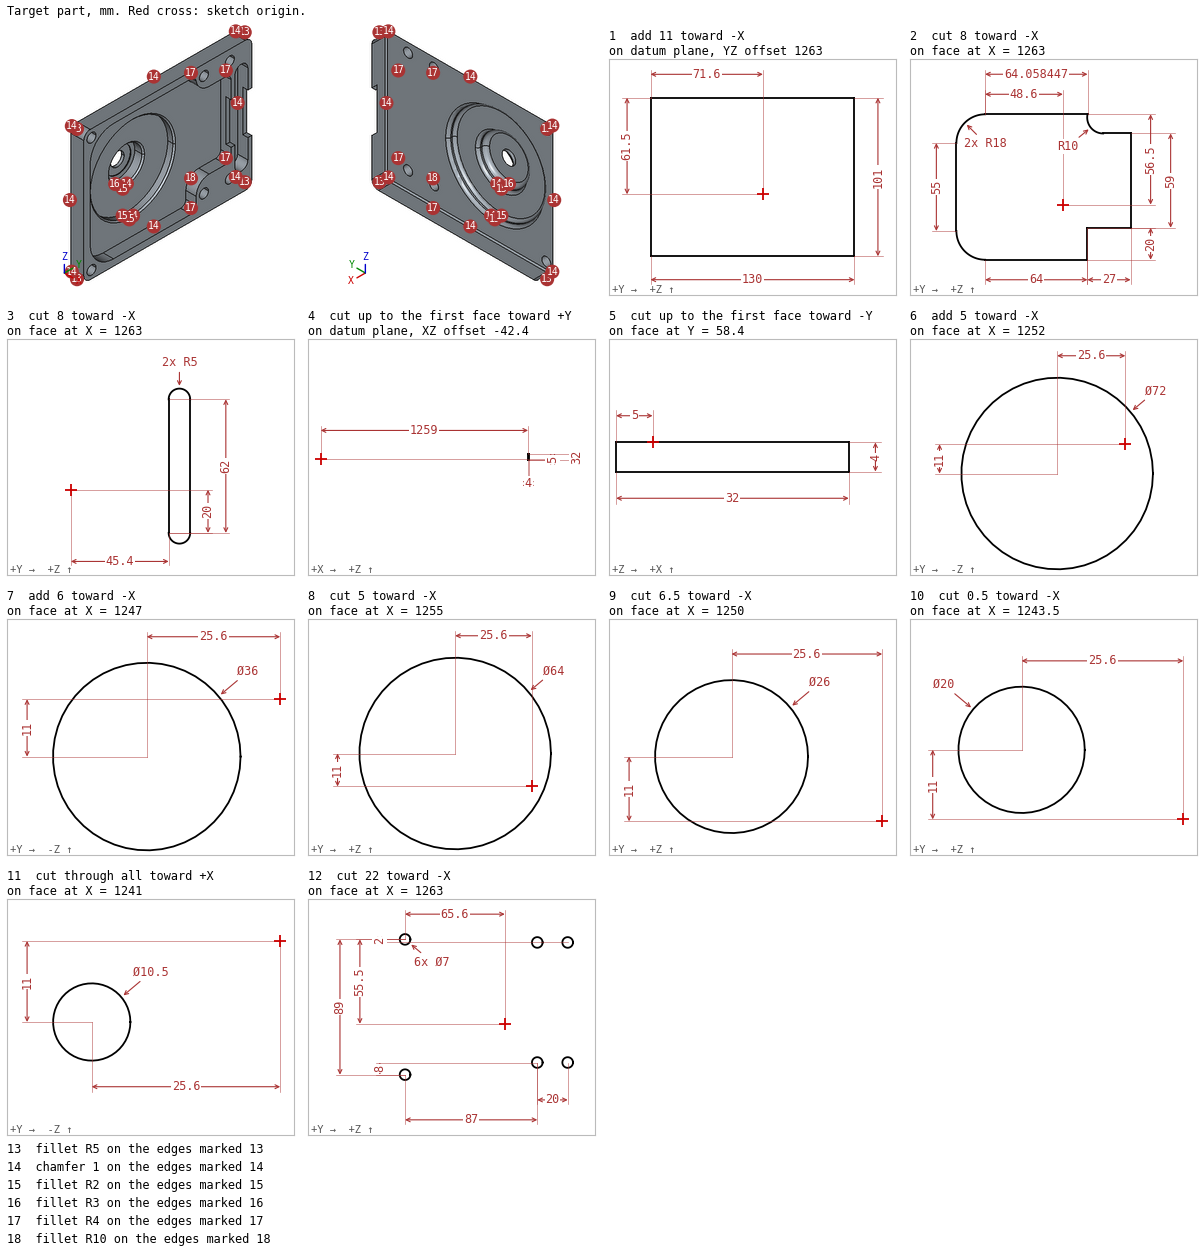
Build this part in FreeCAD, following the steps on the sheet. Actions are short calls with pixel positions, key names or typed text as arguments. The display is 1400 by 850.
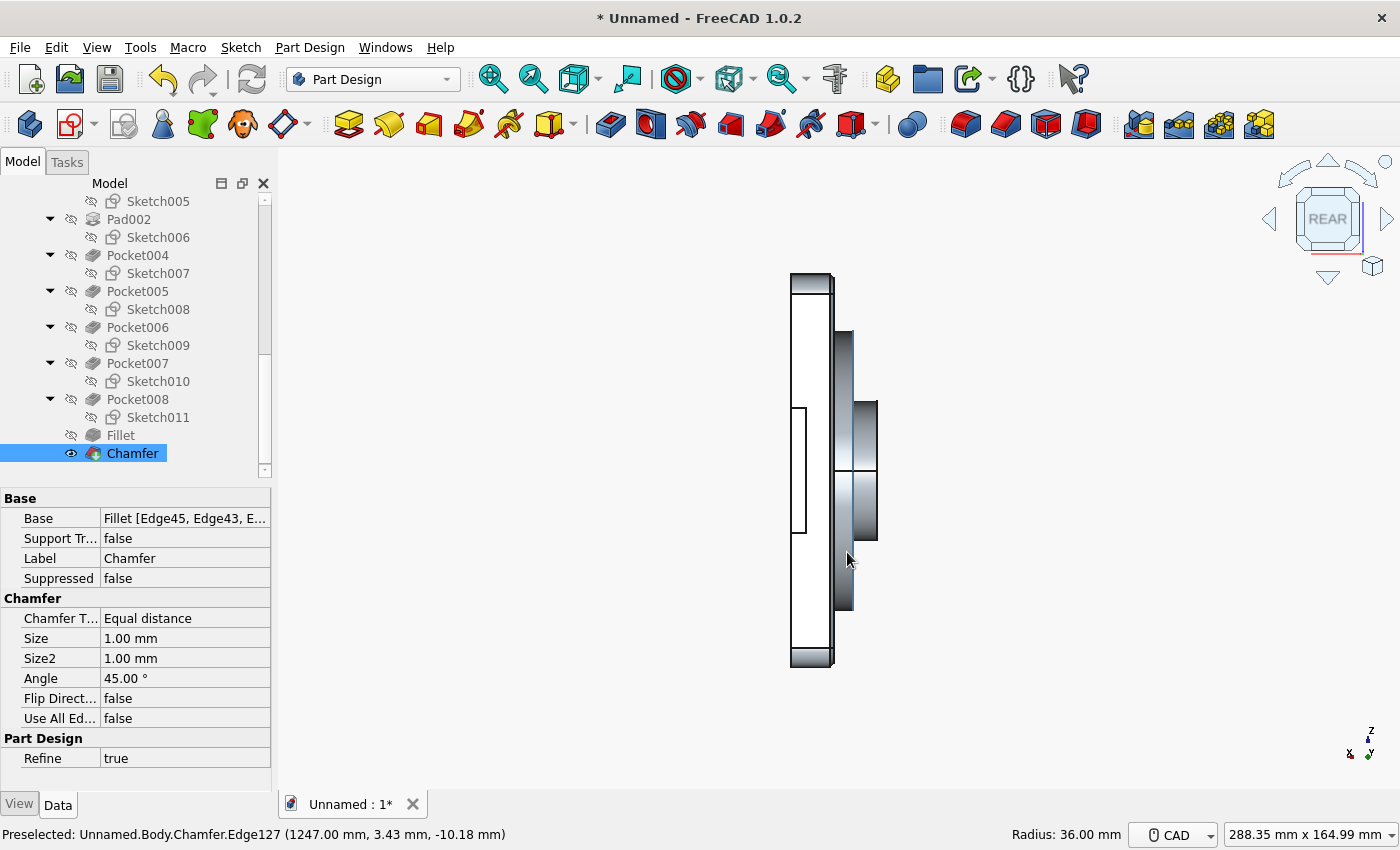
key(6)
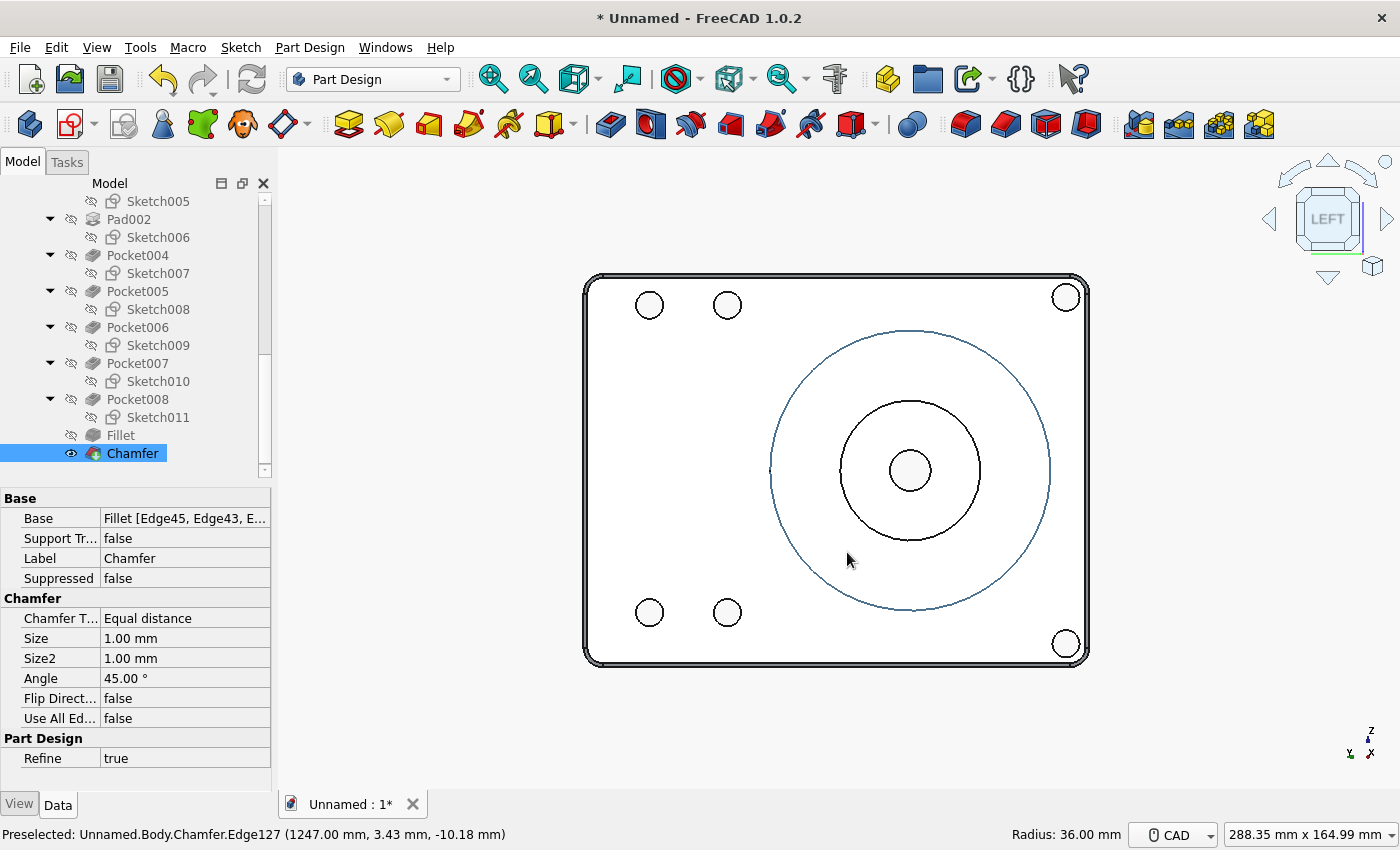
key(v)
key(3)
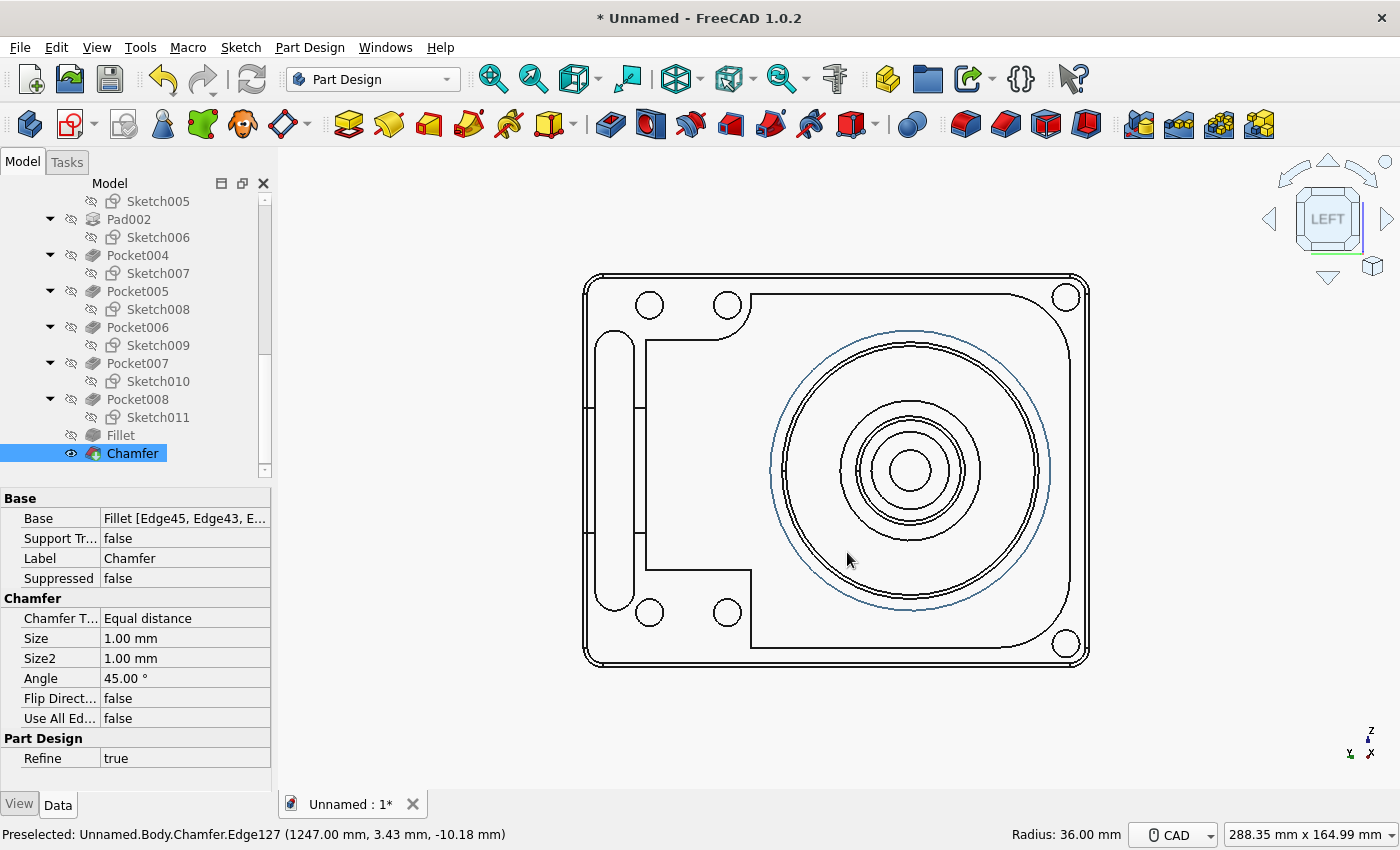
key(0)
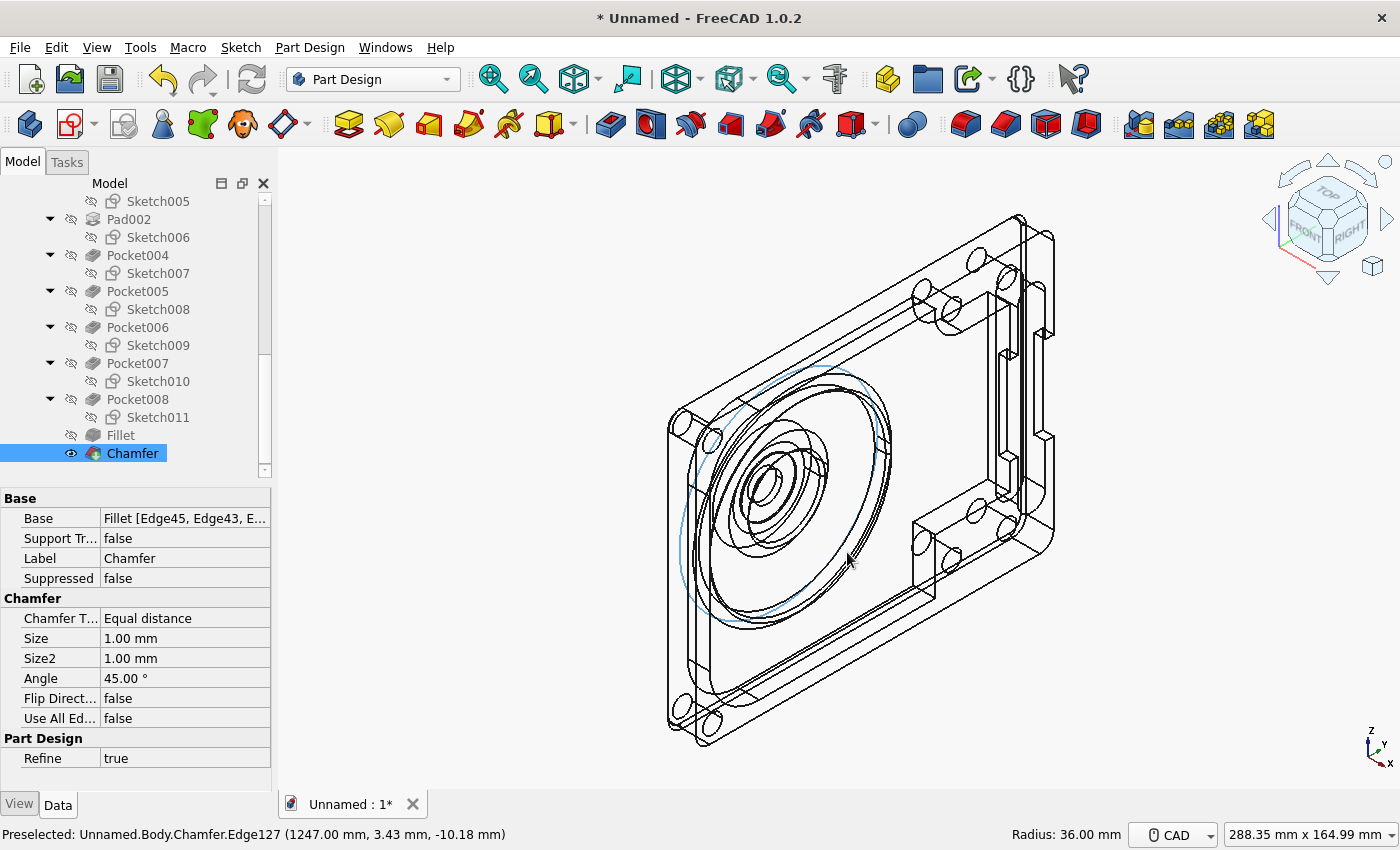
click(864, 380, ctrl)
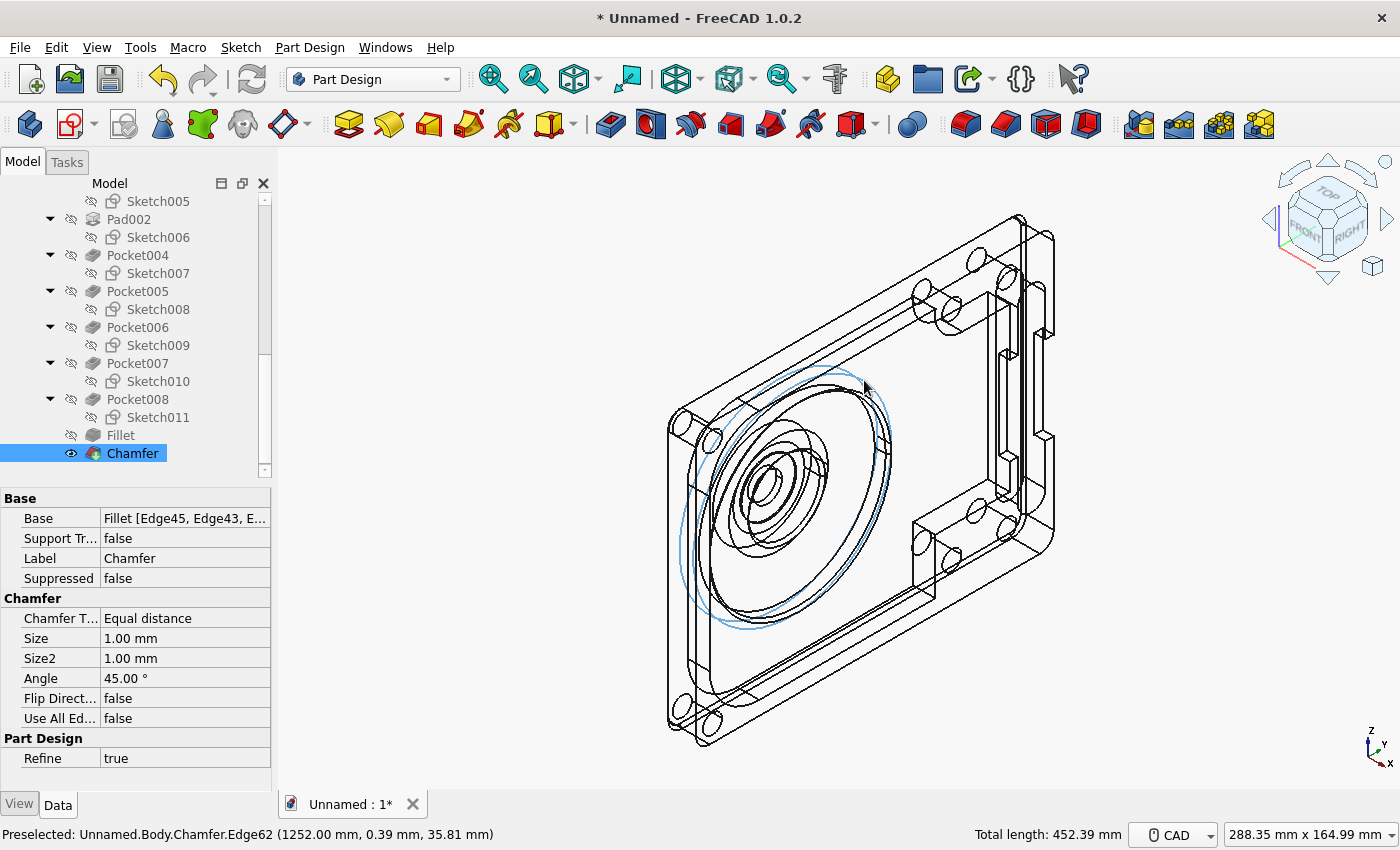
click(729, 521, ctrl)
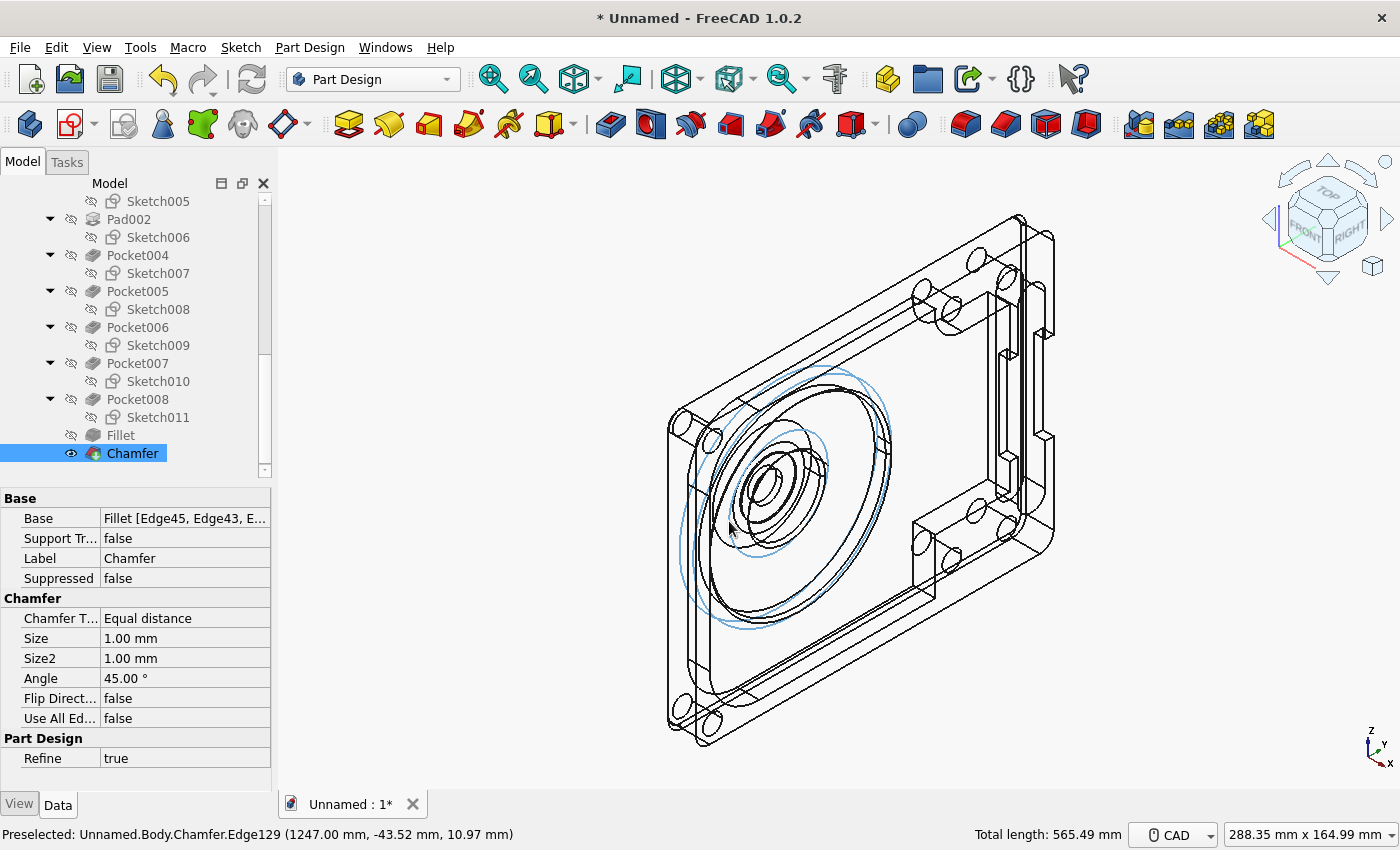
key(v)
key(1)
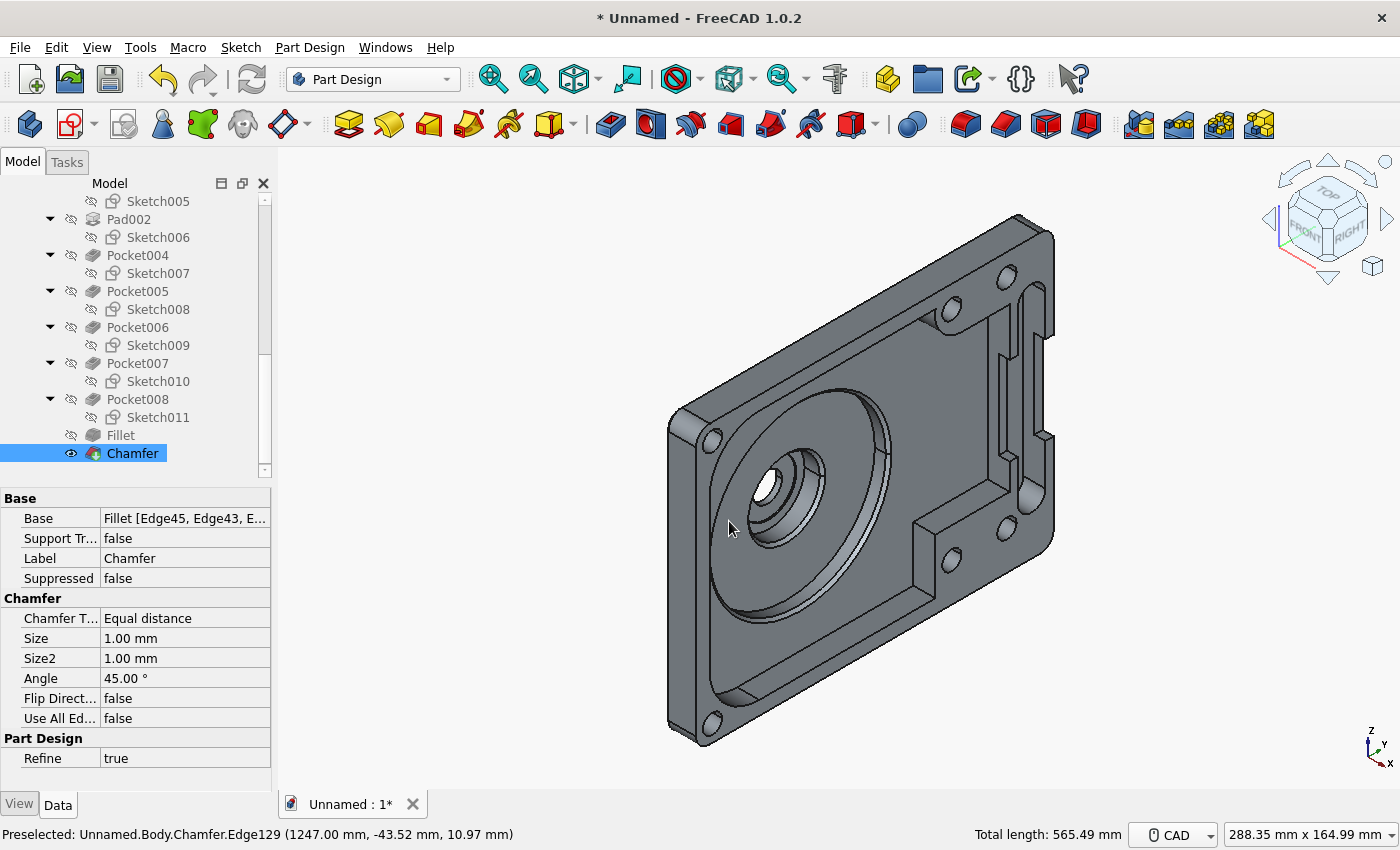
click(966, 124)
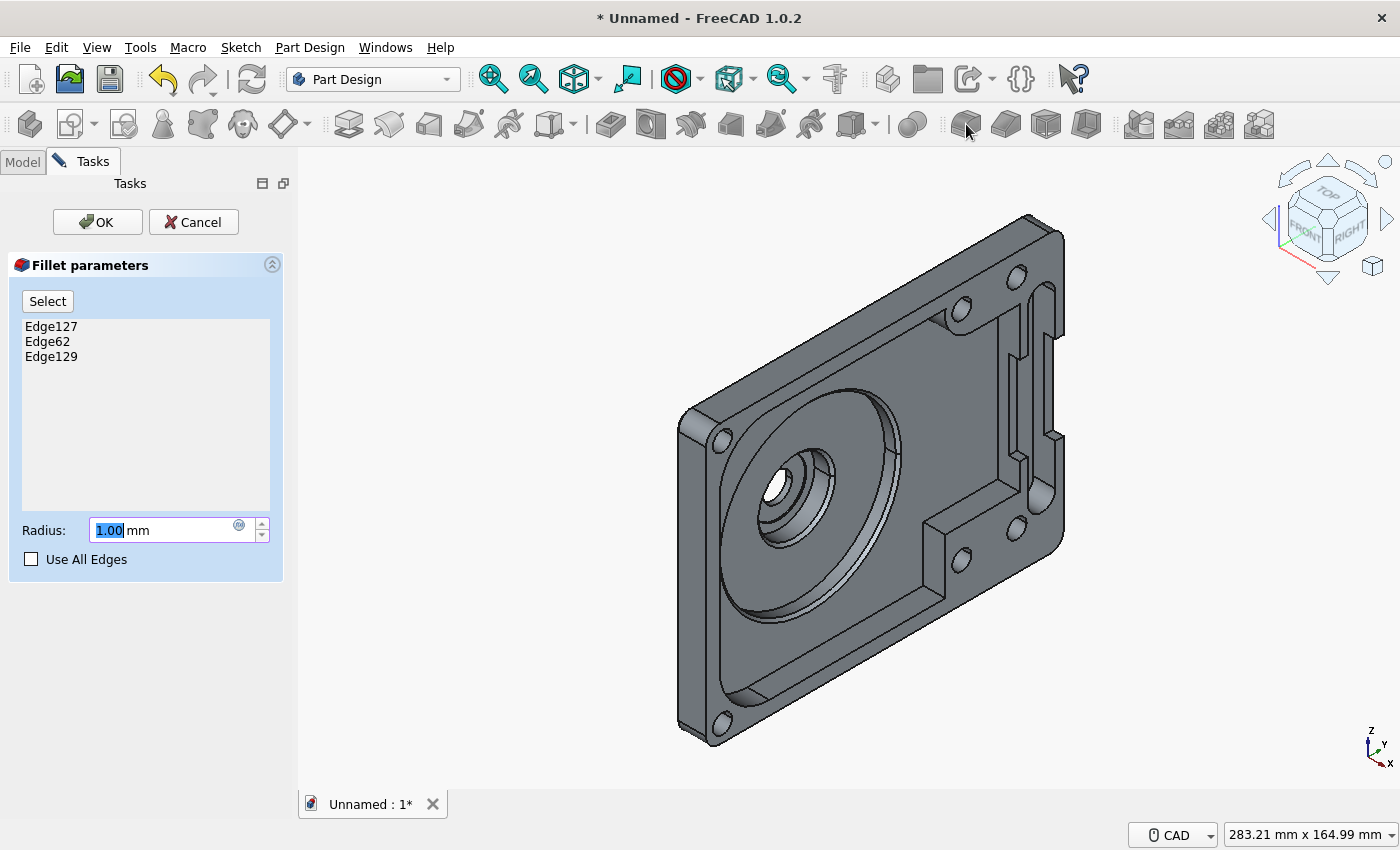
text(2)
key(Tab)